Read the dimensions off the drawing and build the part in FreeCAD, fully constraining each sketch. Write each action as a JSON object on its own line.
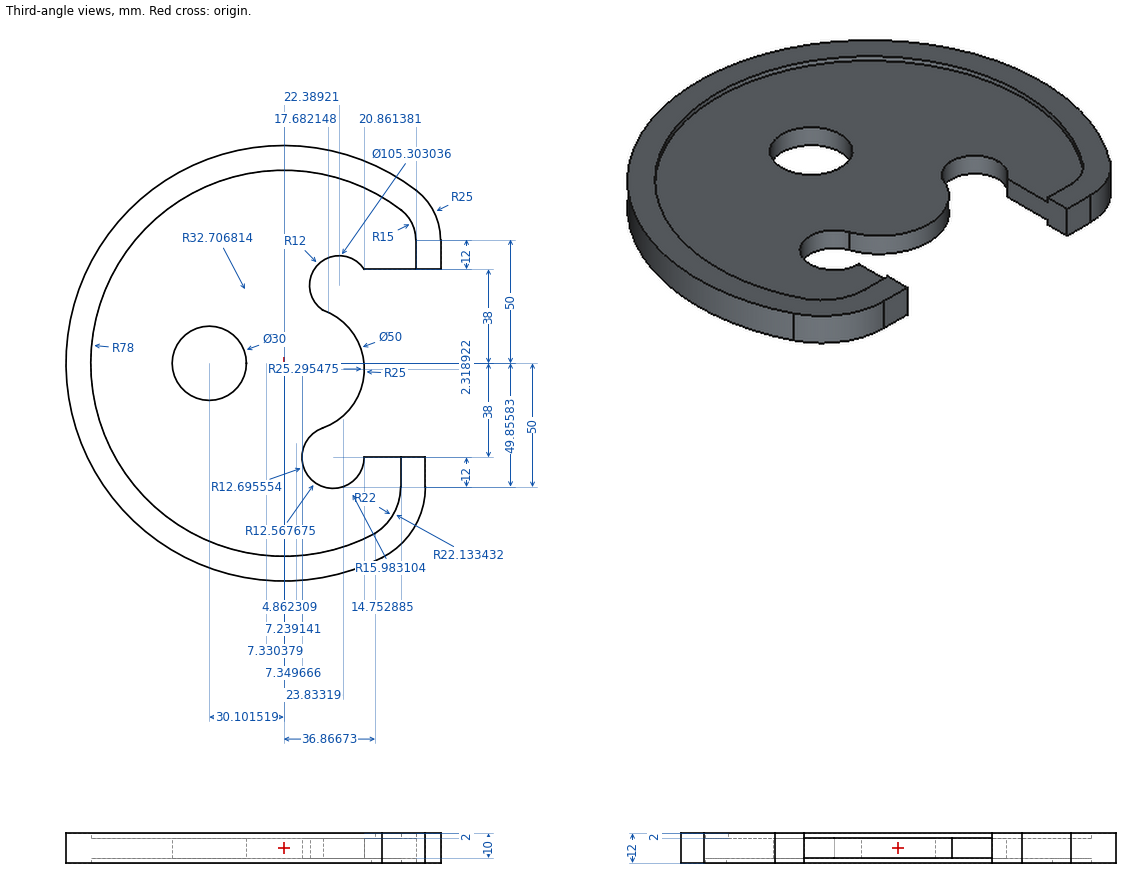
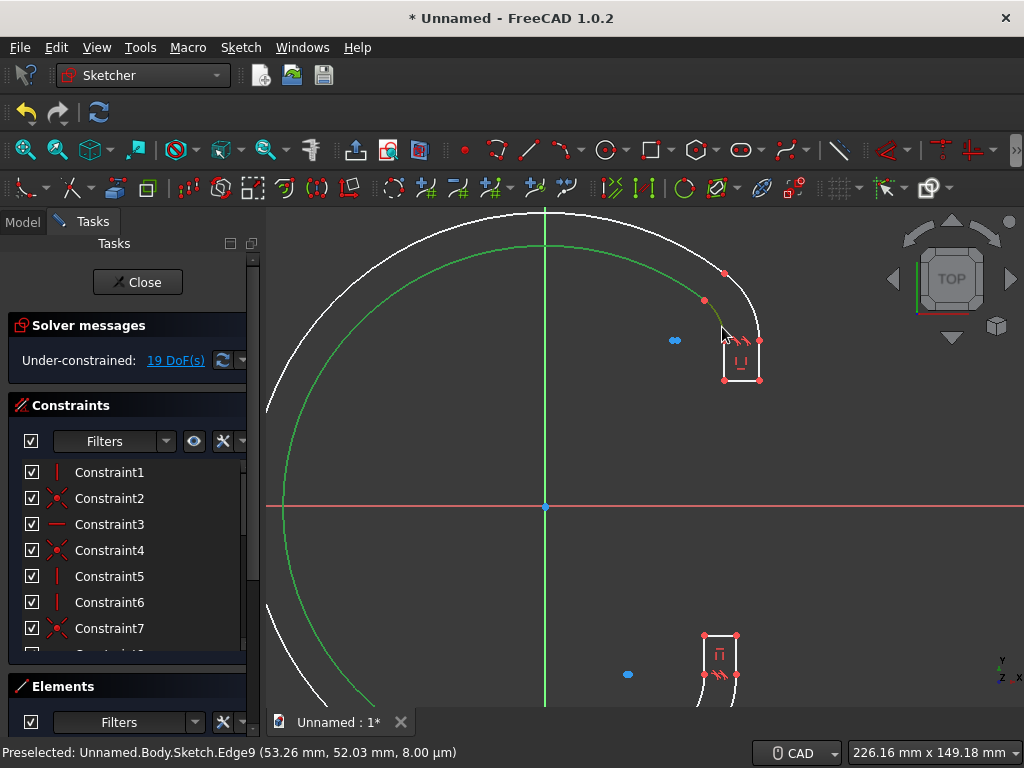
{"action": "key", "text": "t"}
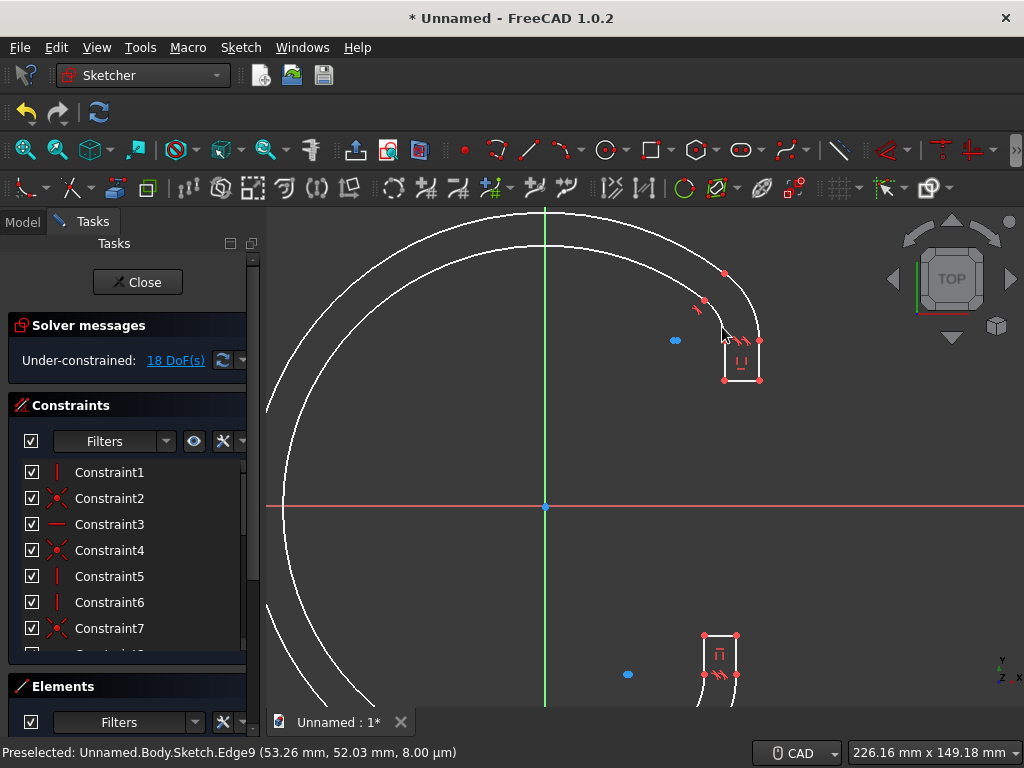
{"action": "left_click", "coordinate": [756, 317]}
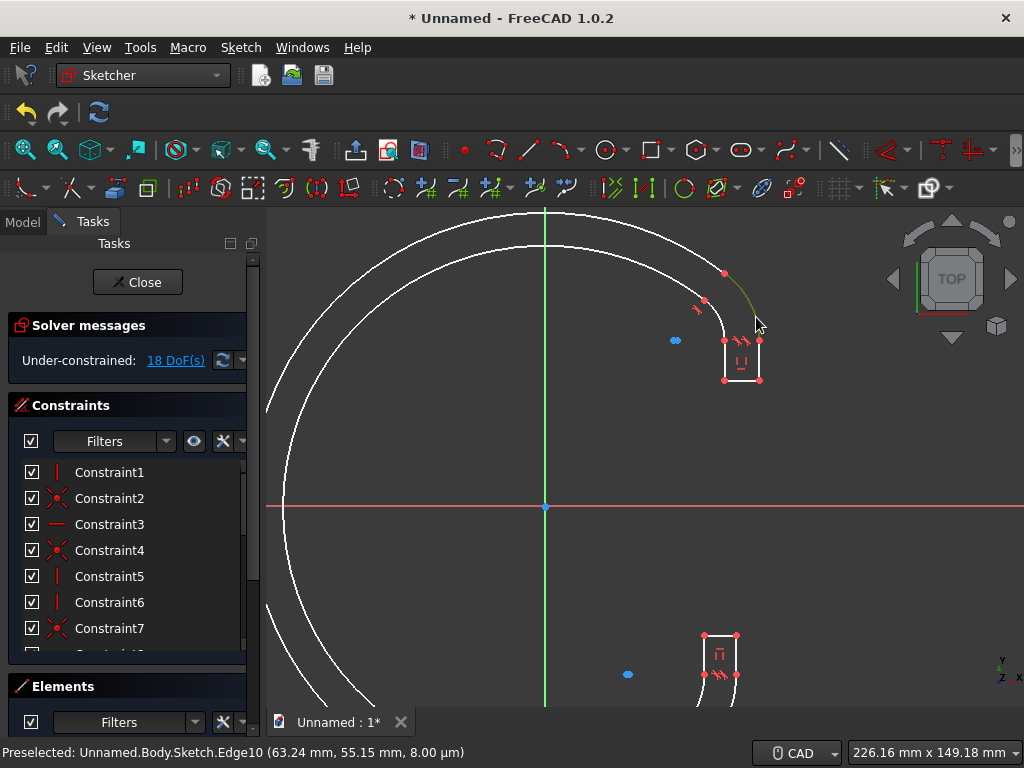
{"action": "left_click", "coordinate": [372, 269]}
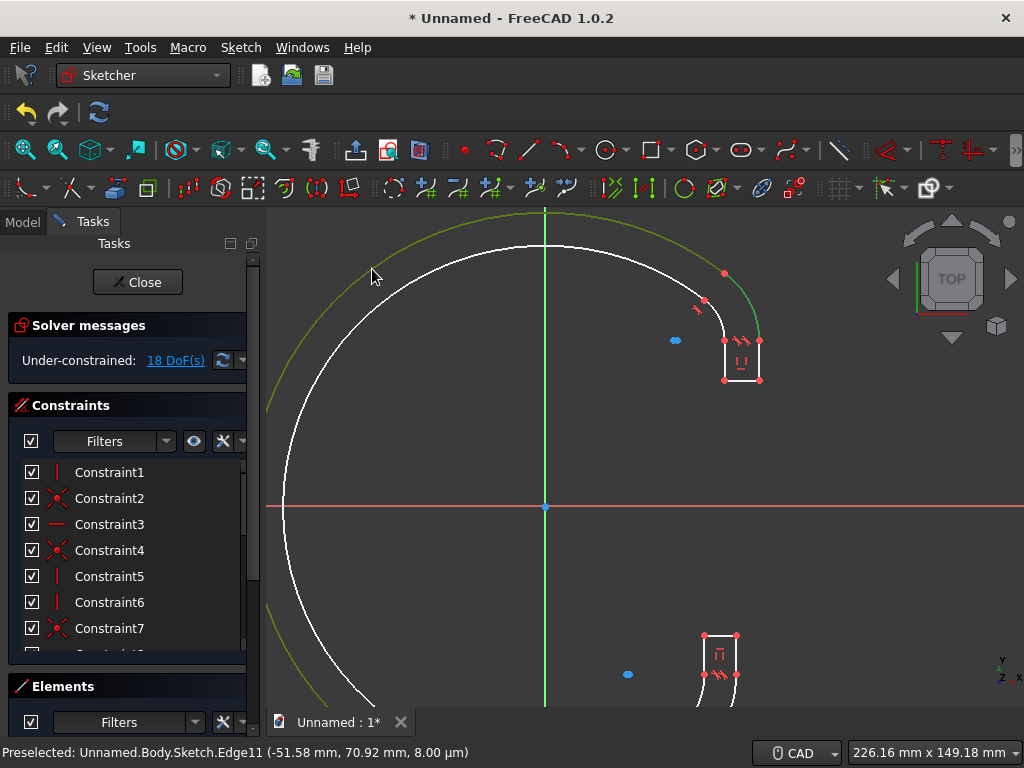
{"action": "key", "text": "t"}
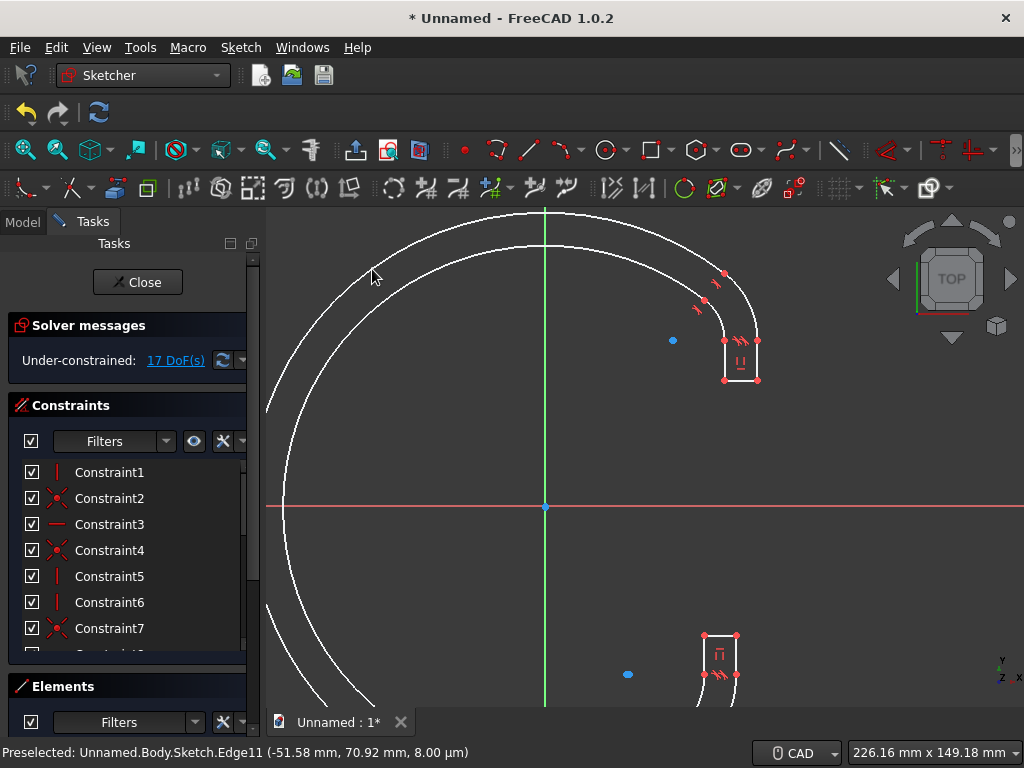
{"action": "left_click", "coordinate": [372, 269]}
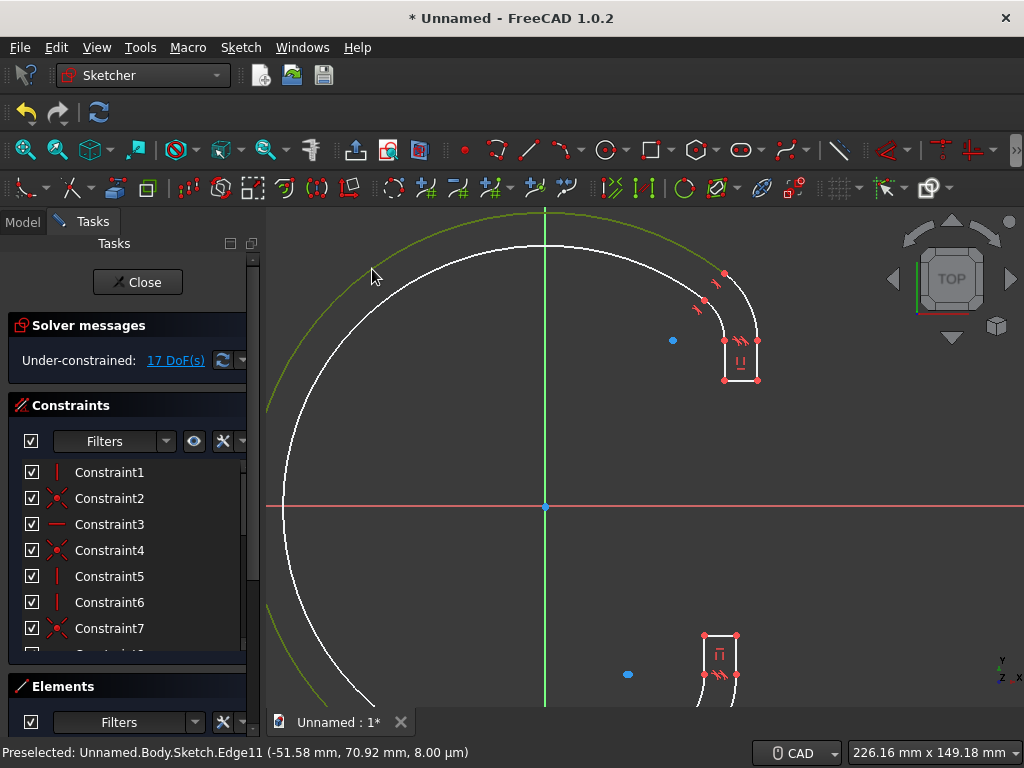
{"action": "scroll", "coordinate": [723, 327], "scroll_direction": "down", "scroll_amount": 2}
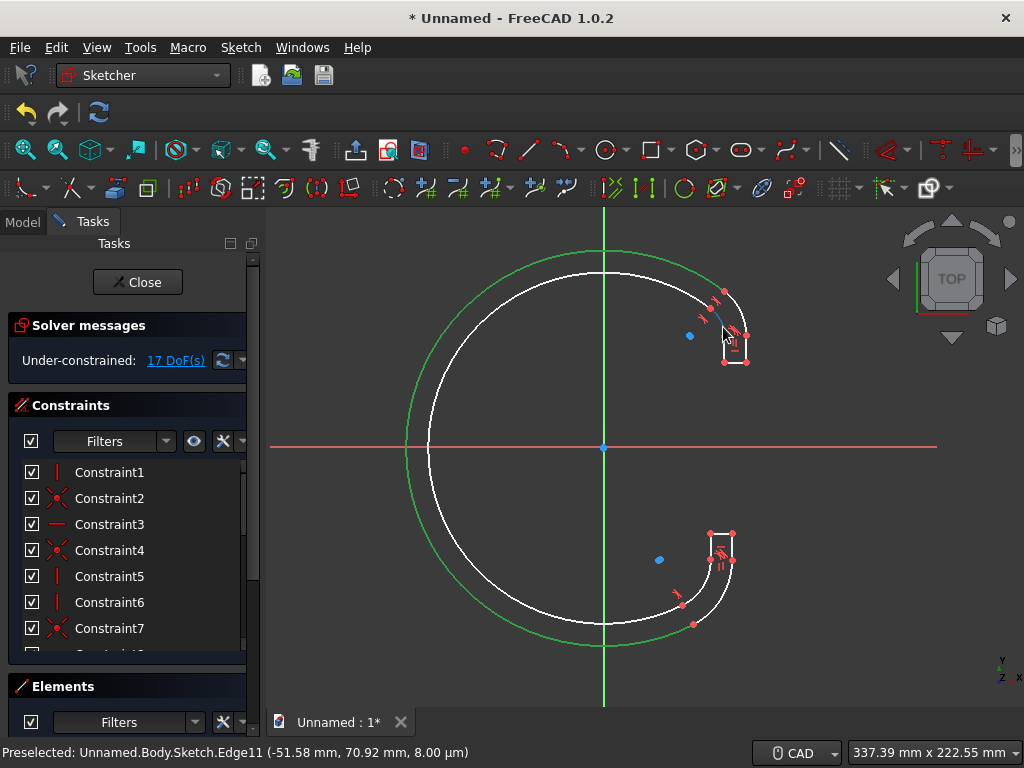
{"action": "left_click", "coordinate": [712, 611]}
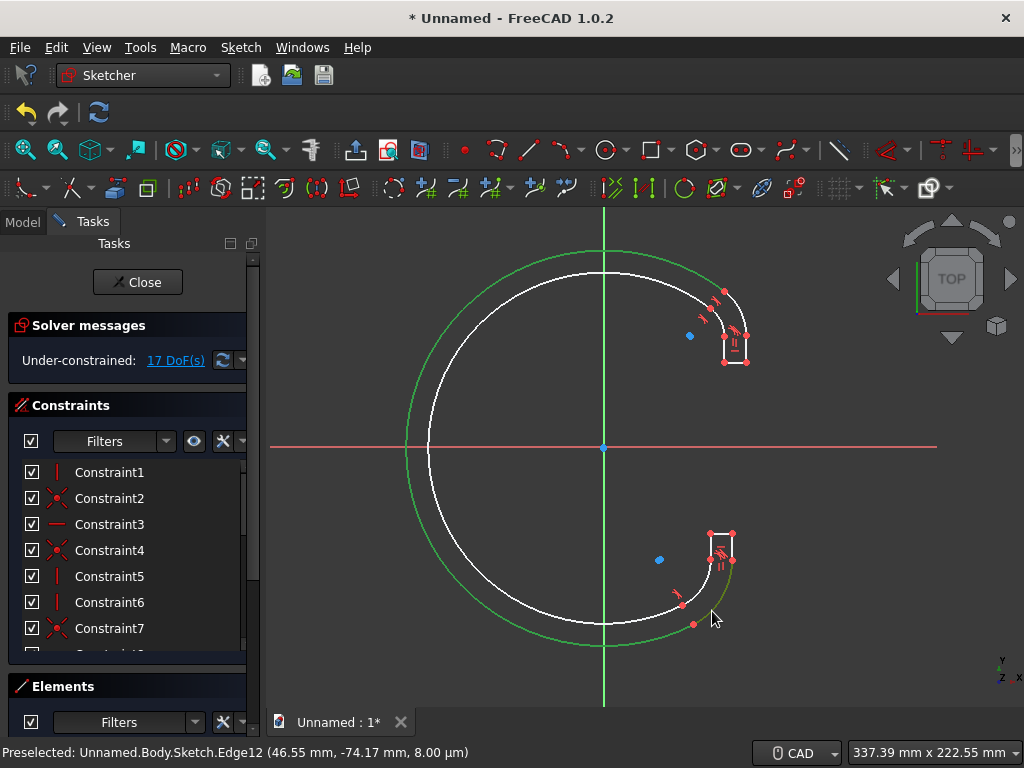
{"action": "key", "text": "t"}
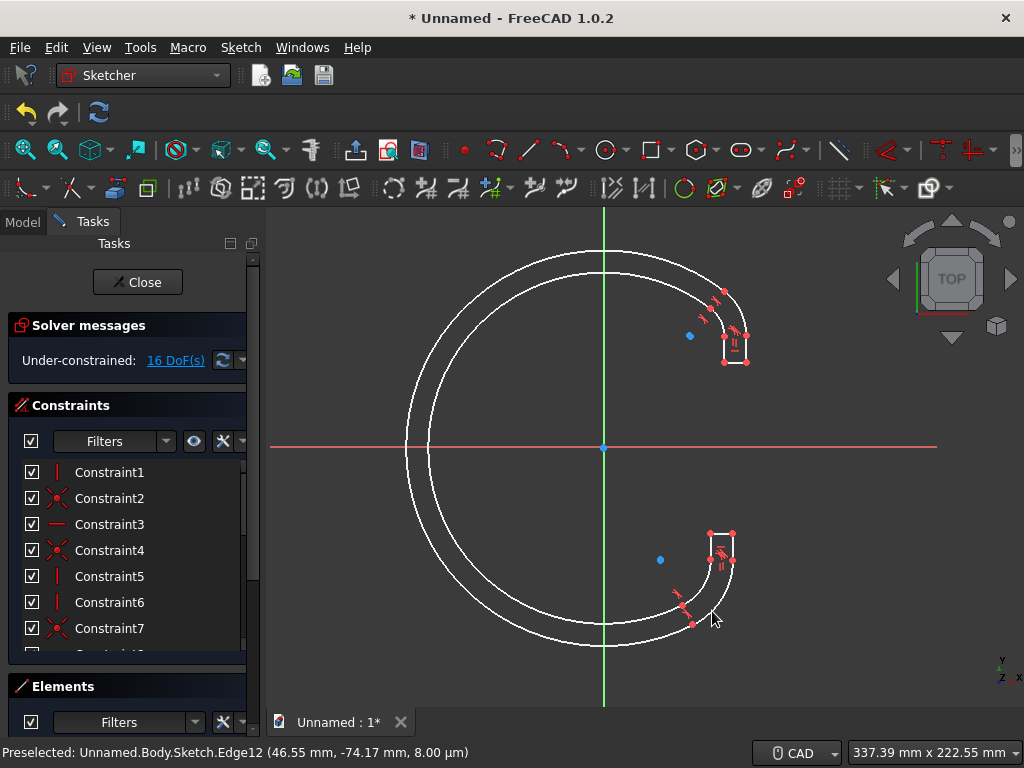
{"action": "scroll", "coordinate": [723, 327], "scroll_direction": "up", "scroll_amount": 2}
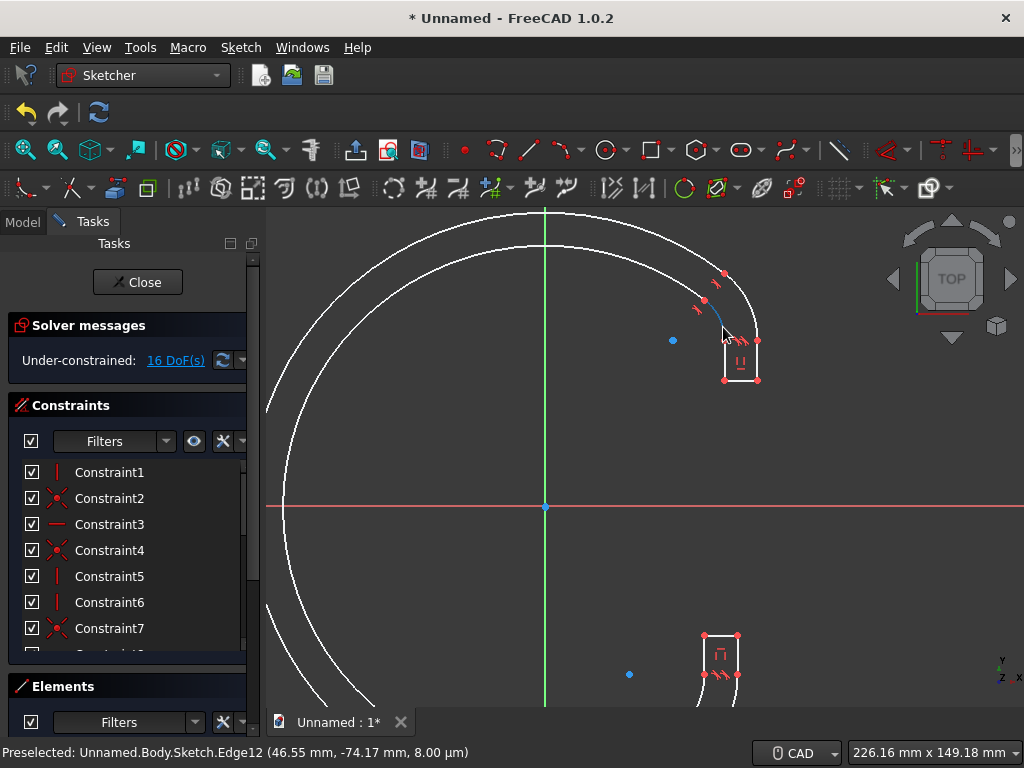
{"action": "left_click", "coordinate": [723, 327]}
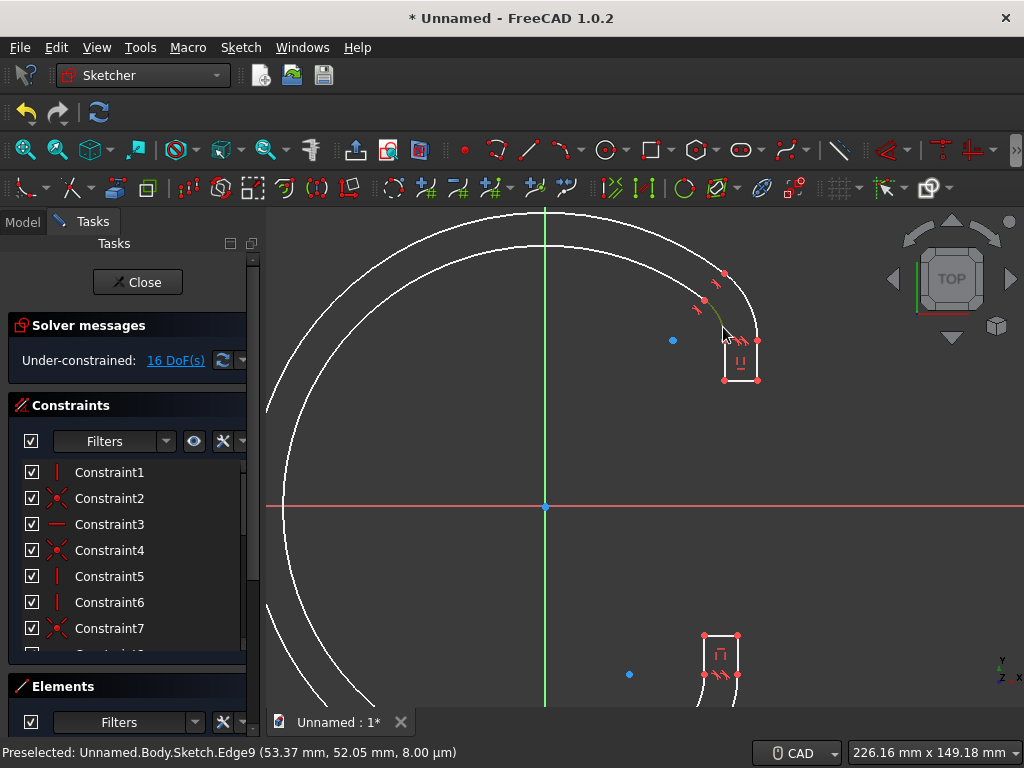
{"action": "left_click", "coordinate": [754, 317]}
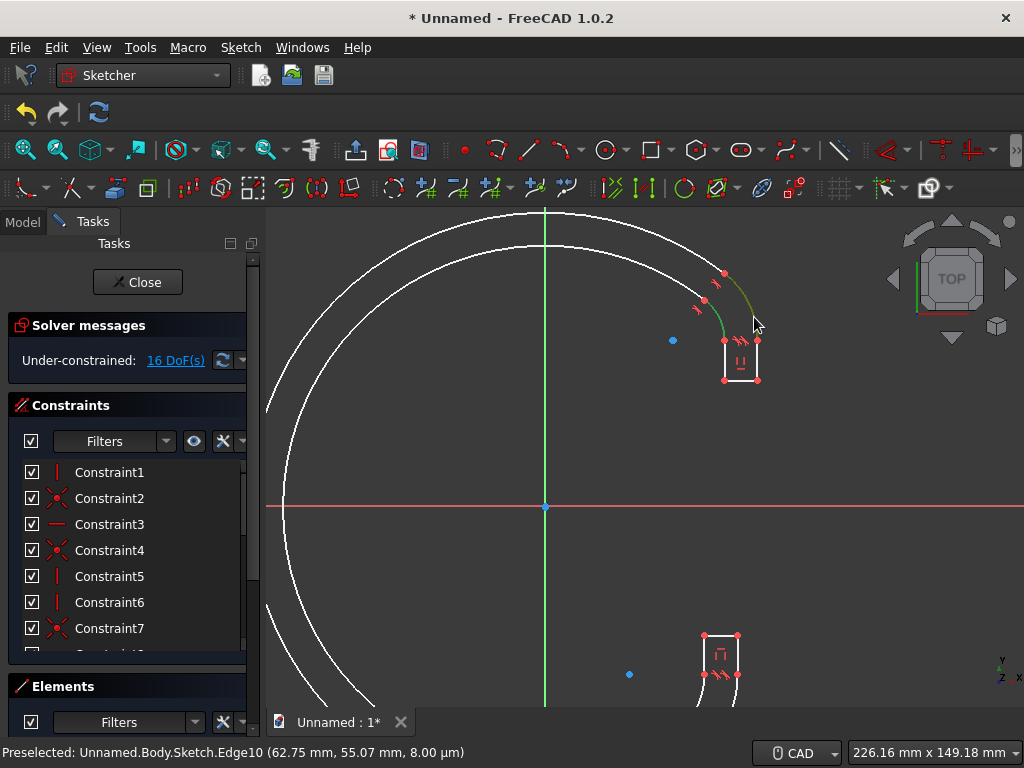
{"action": "key", "text": "c"}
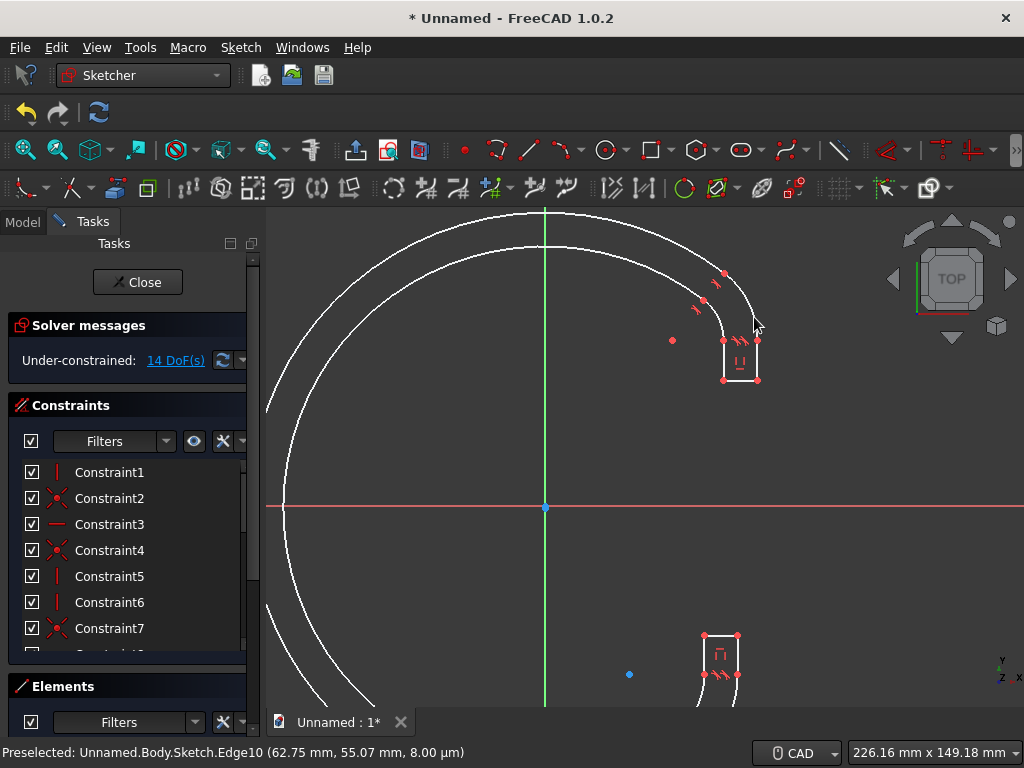
{"action": "left_click", "coordinate": [392, 296]}